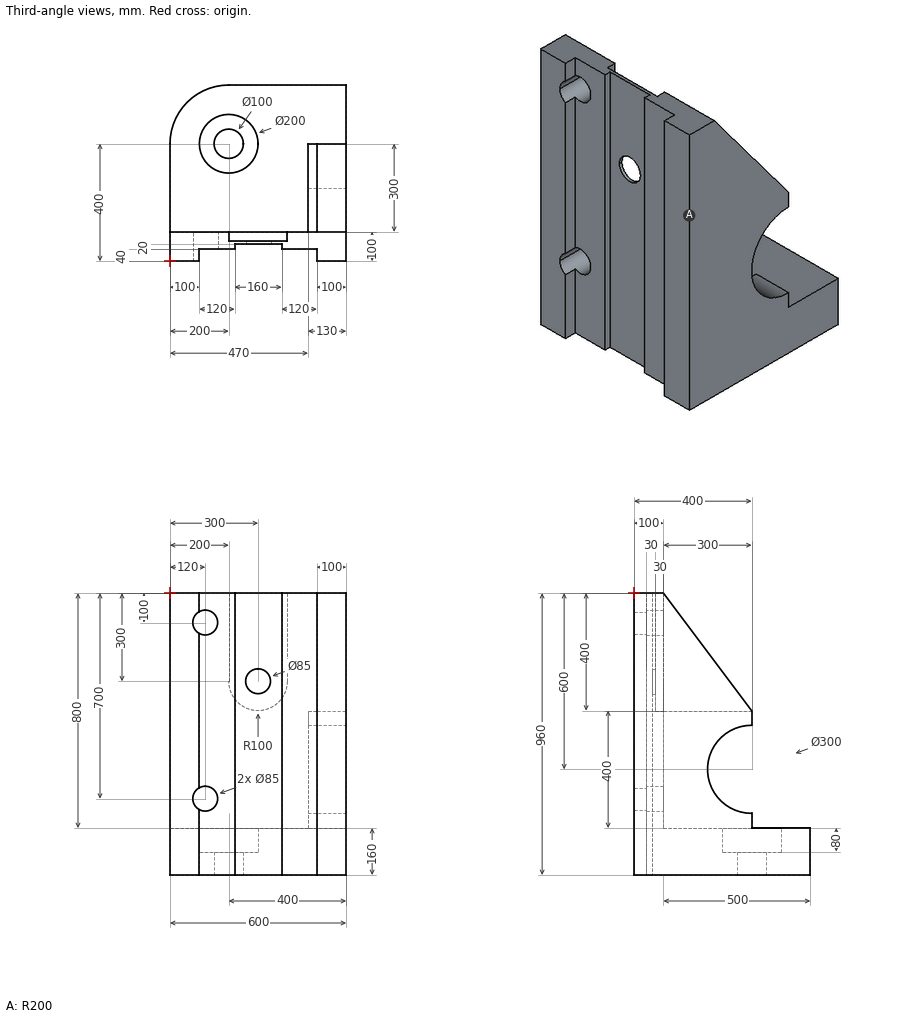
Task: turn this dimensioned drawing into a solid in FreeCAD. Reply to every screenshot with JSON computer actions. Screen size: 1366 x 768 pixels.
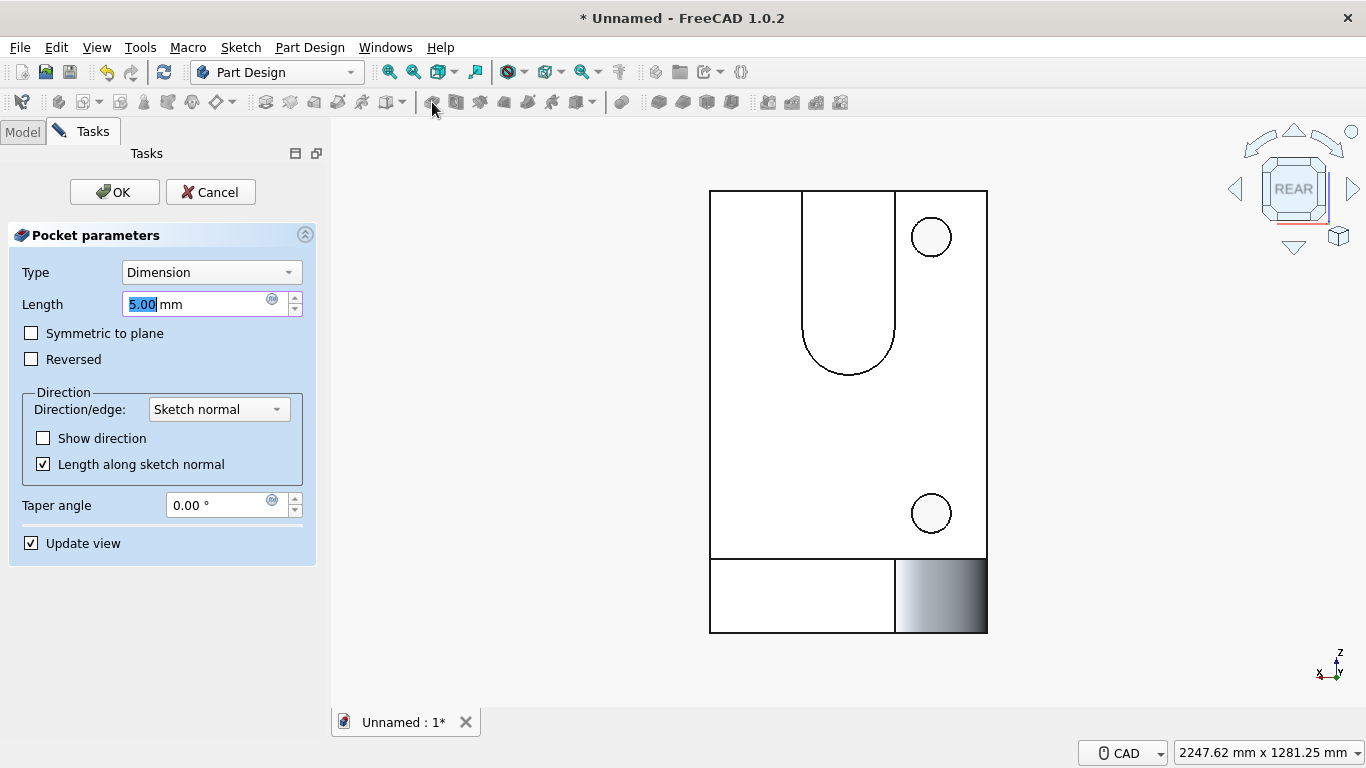
{"action": "type", "text": "30"}
{"action": "key", "text": "Tab"}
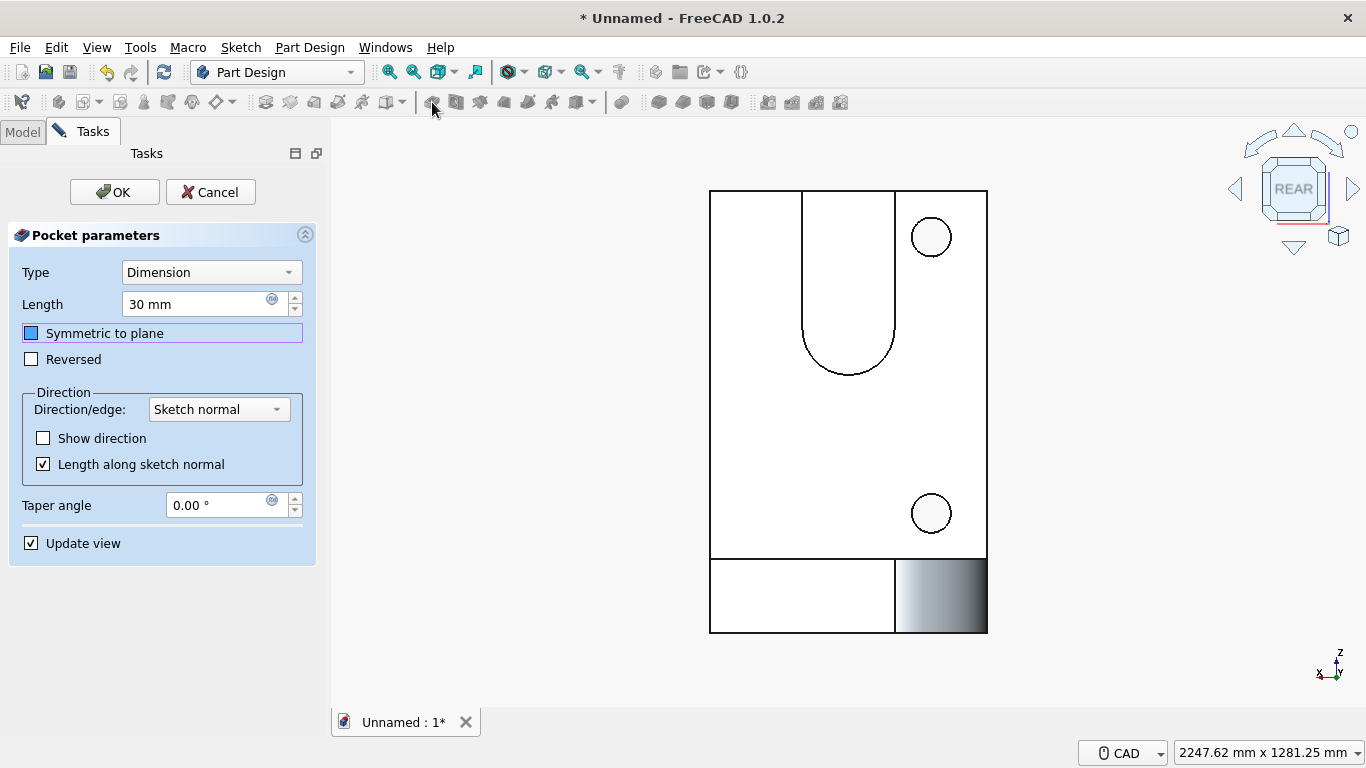
{"action": "left_click", "coordinate": [115, 192]}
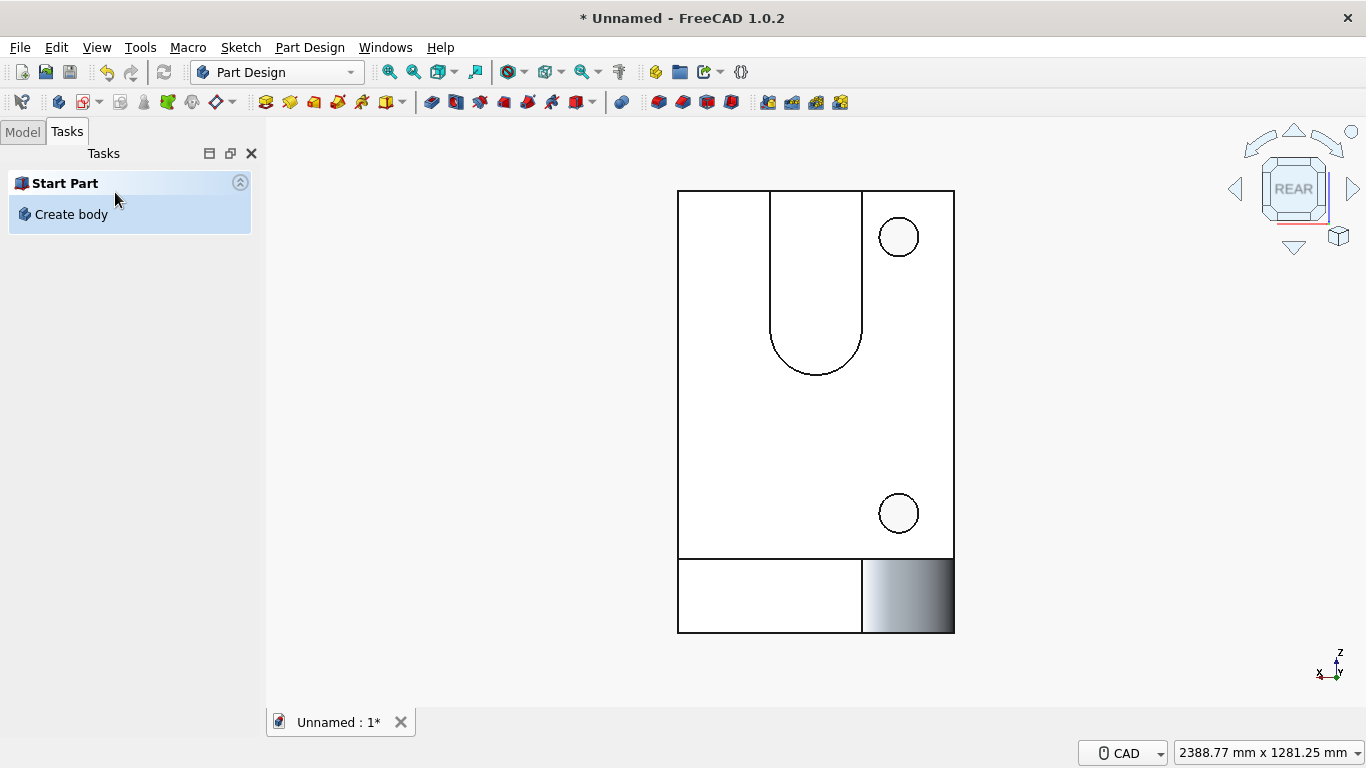
{"action": "left_click", "coordinate": [816, 256]}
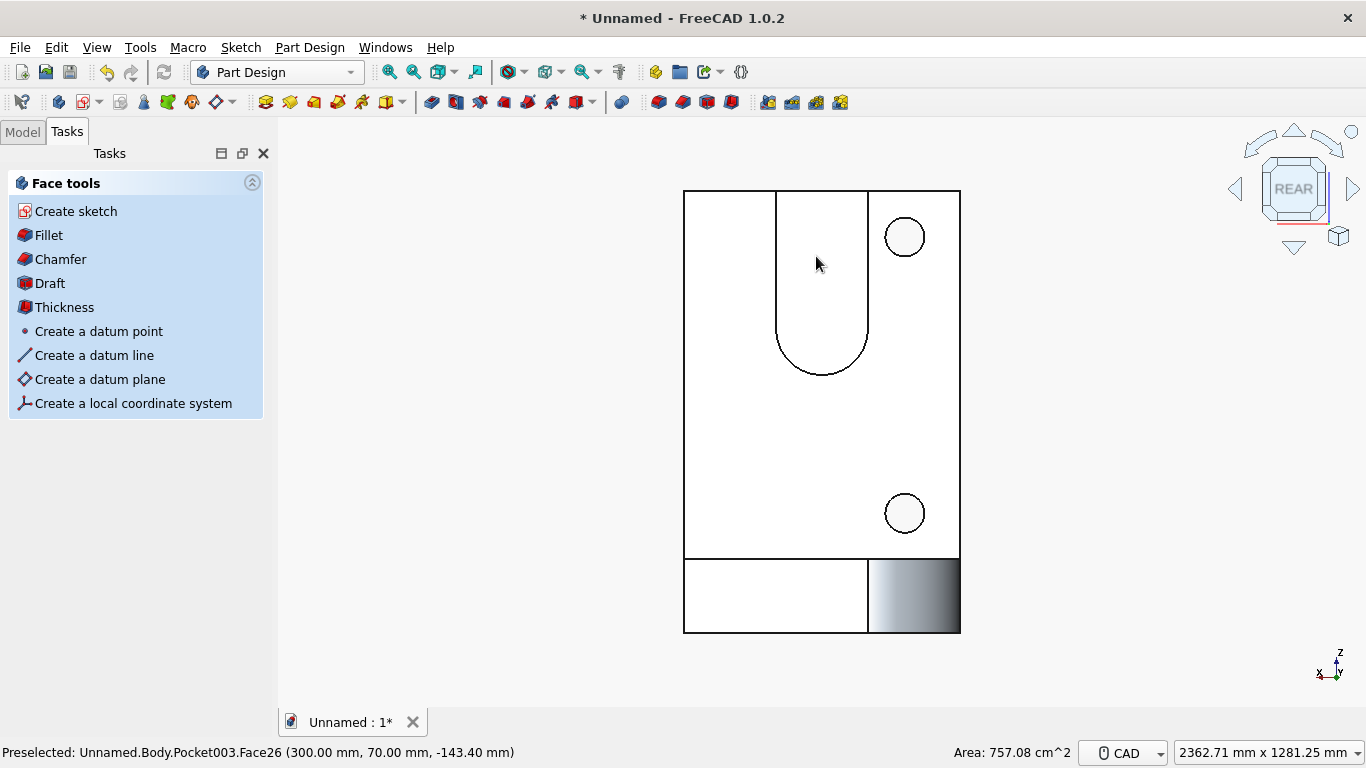
{"action": "left_click", "coordinate": [84, 102]}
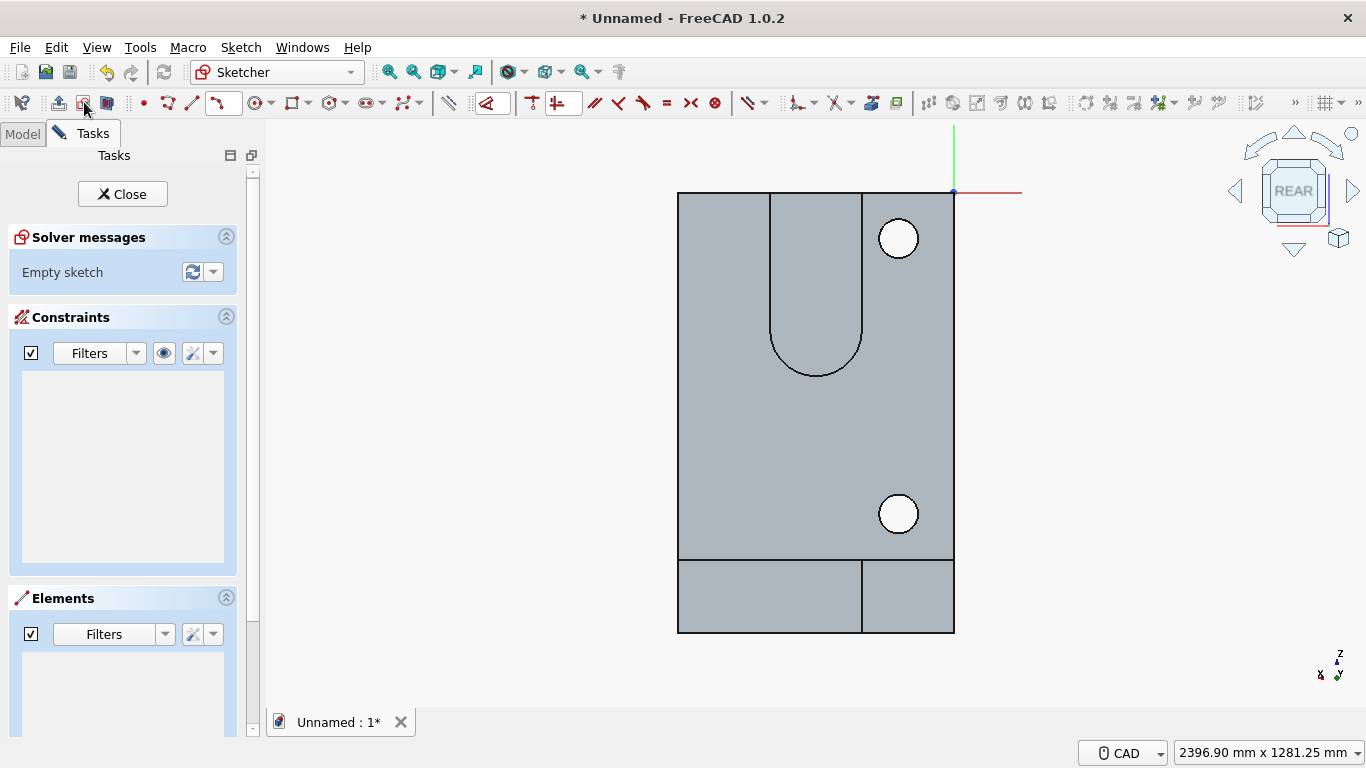
{"action": "left_click", "coordinate": [108, 104]}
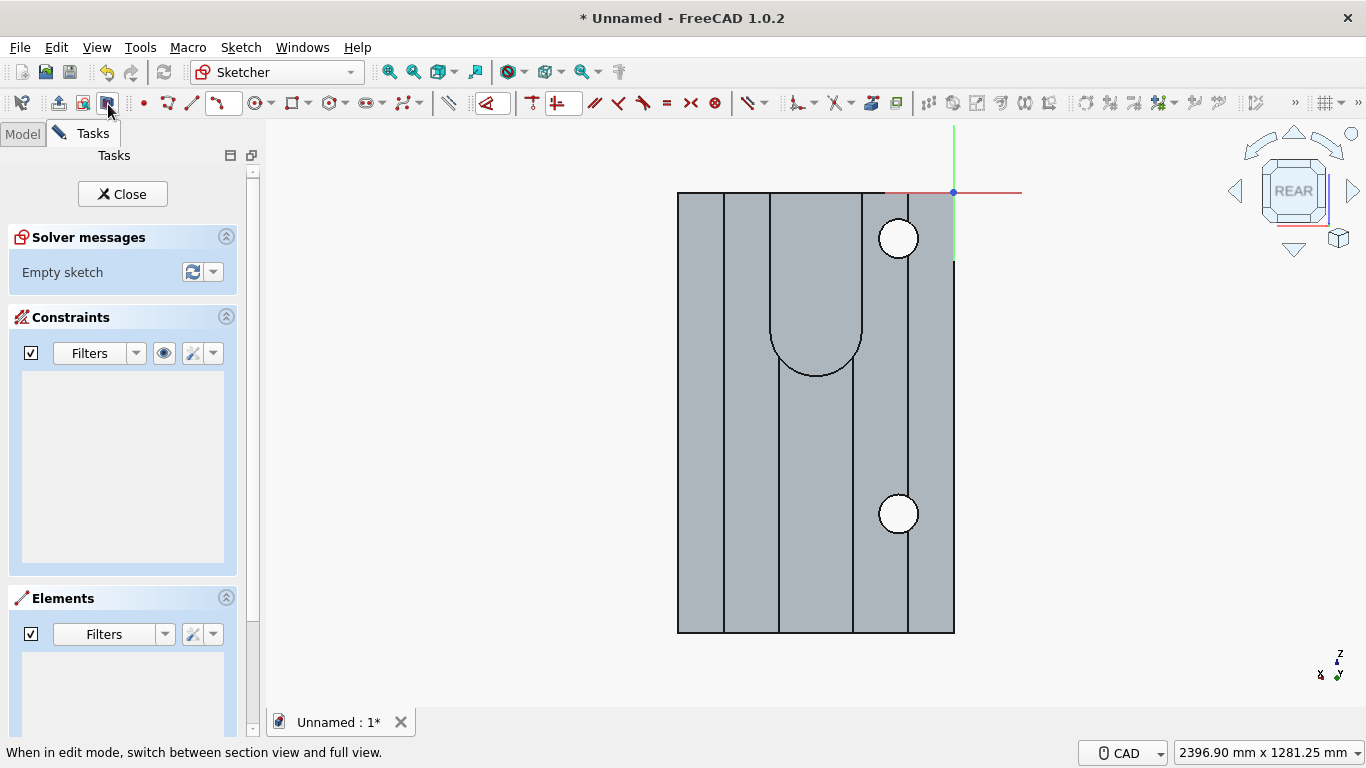
{"action": "scroll", "coordinate": [825, 320], "scroll_direction": "up", "scroll_amount": 11}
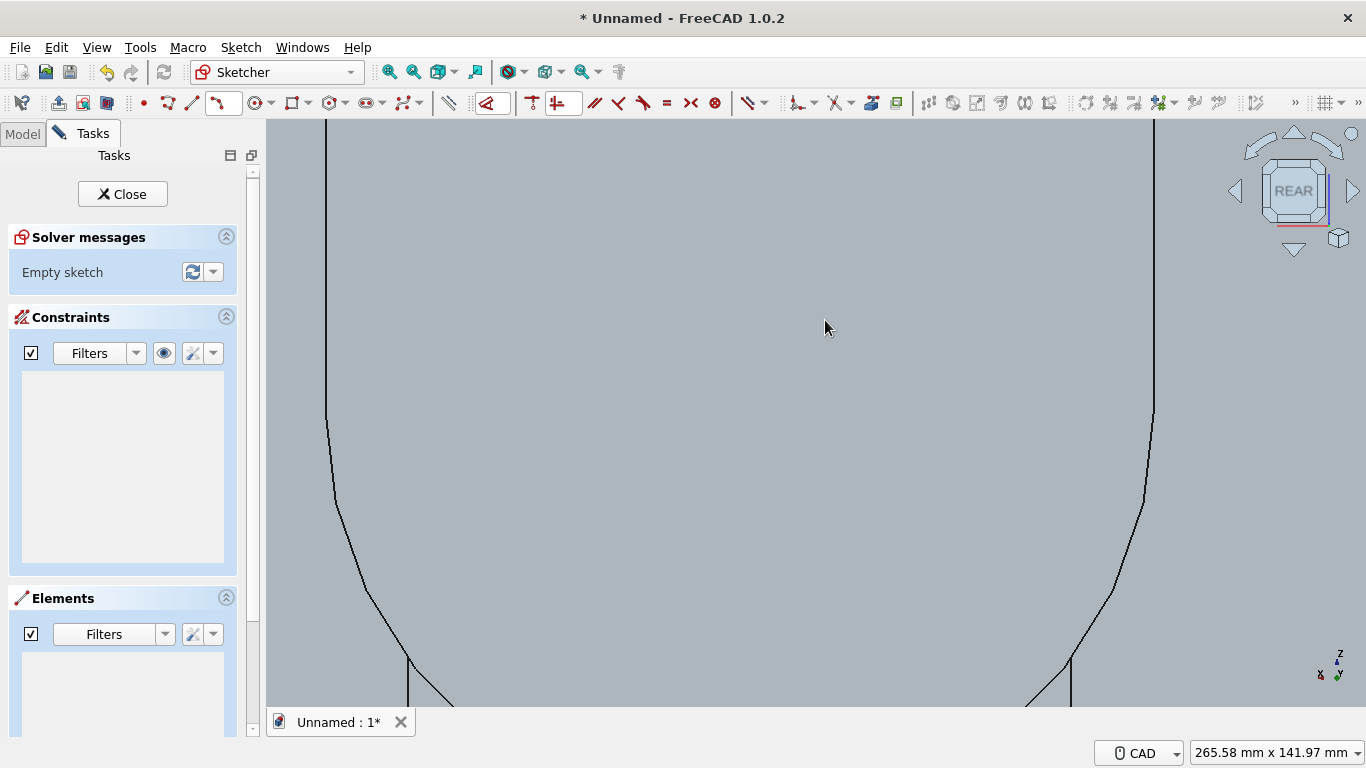
{"action": "left_click", "coordinate": [256, 104]}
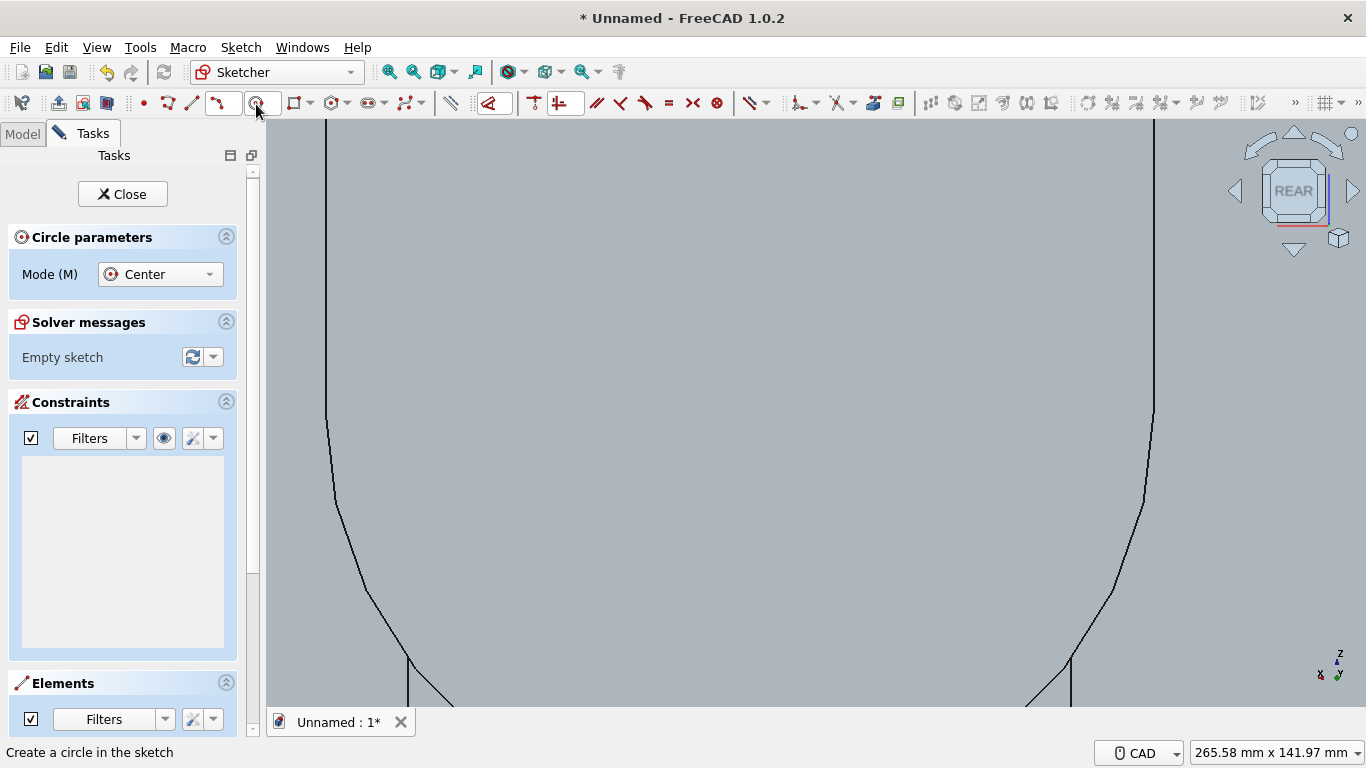
{"action": "left_click", "coordinate": [740, 411]}
{"action": "left_click", "coordinate": [864, 287]}
{"action": "key", "text": "Escape"}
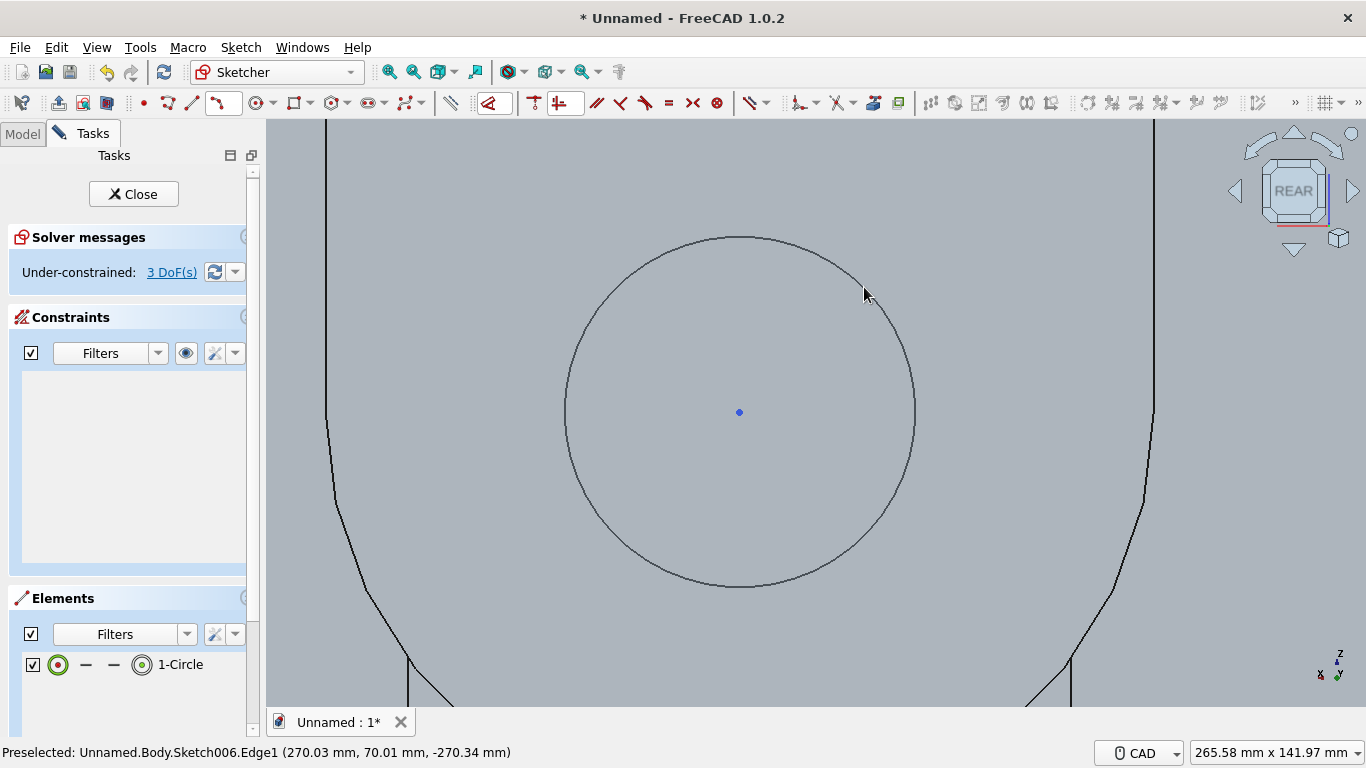
{"action": "left_click", "coordinate": [864, 288]}